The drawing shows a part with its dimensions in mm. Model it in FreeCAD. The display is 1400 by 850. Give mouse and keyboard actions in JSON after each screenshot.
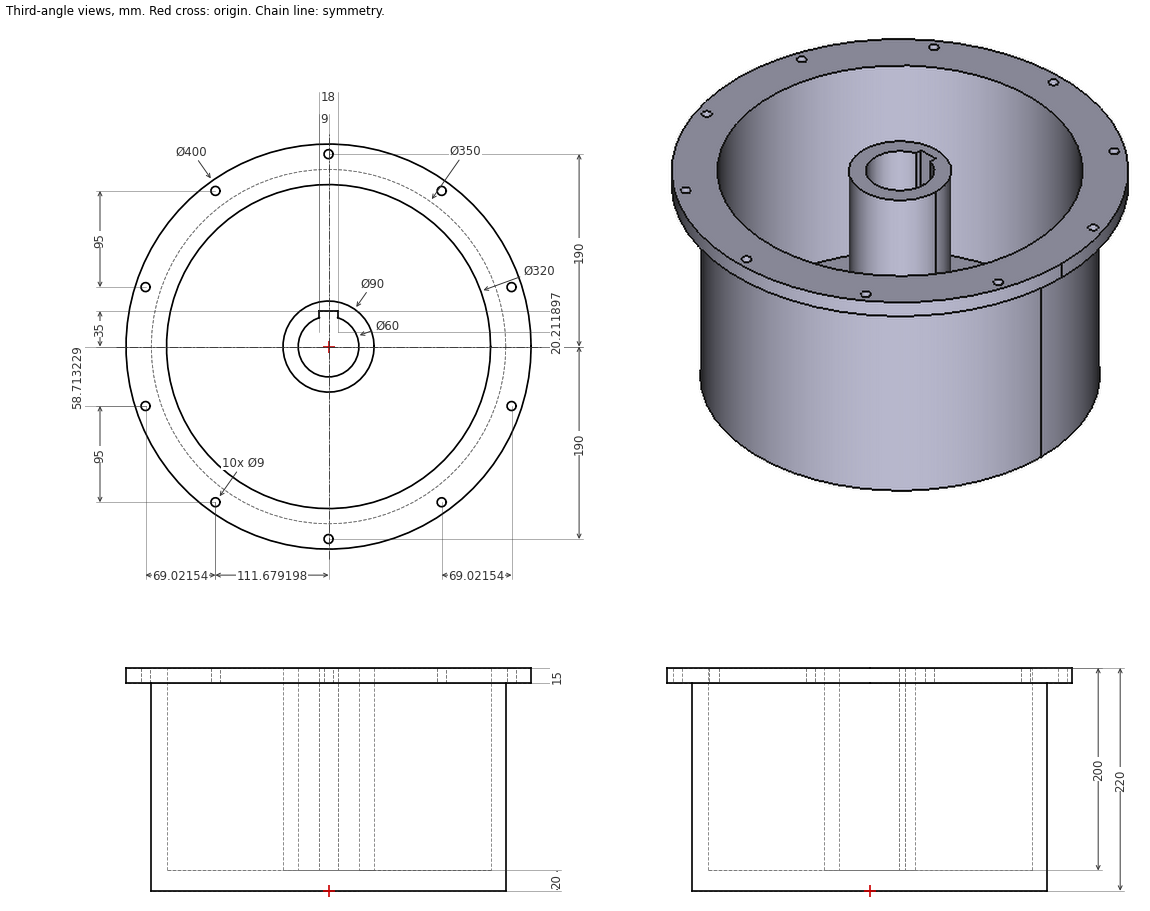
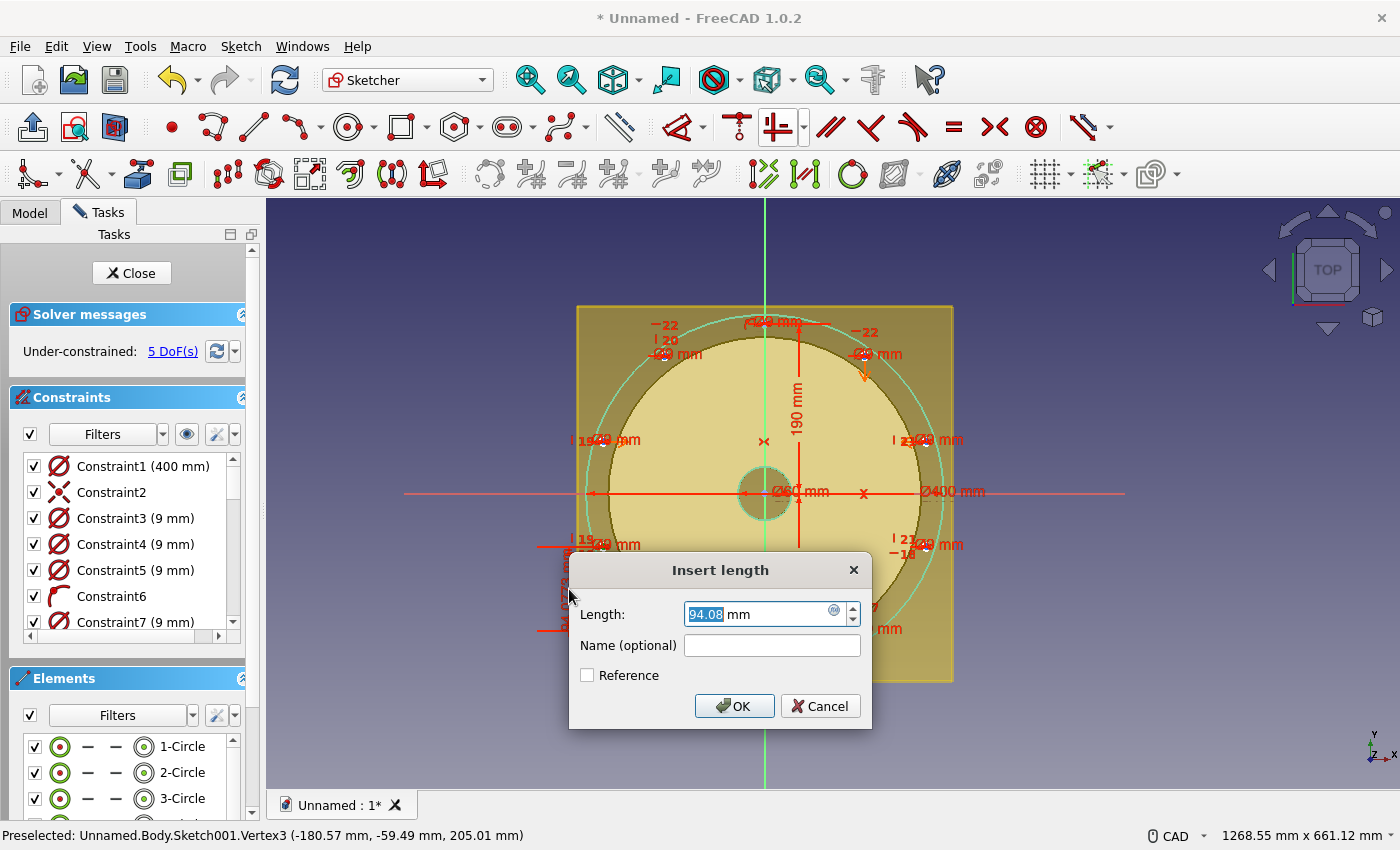
{"action": "type", "text": "95"}
{"action": "key", "text": "Return"}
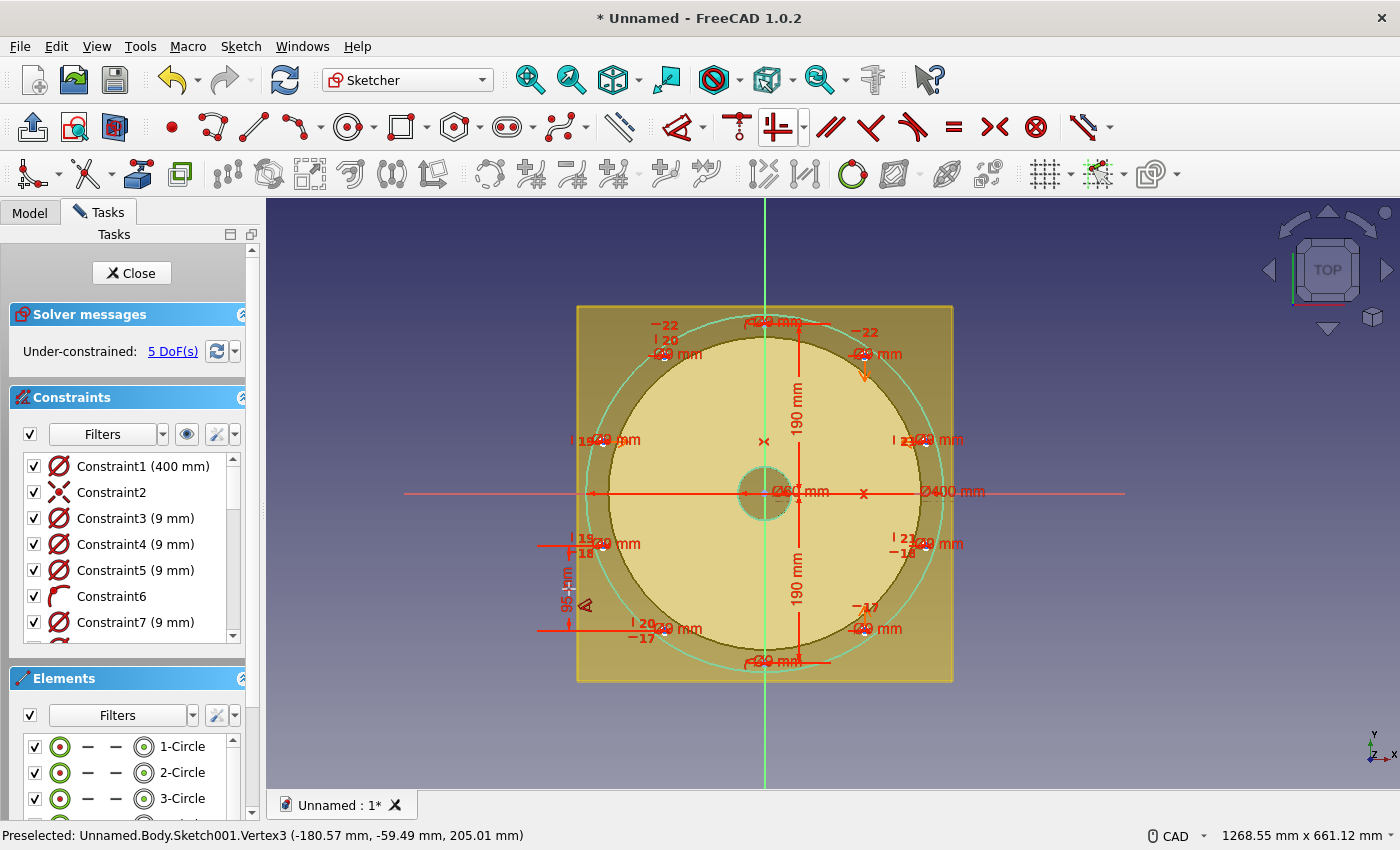
{"action": "left_click", "coordinate": [603, 442]}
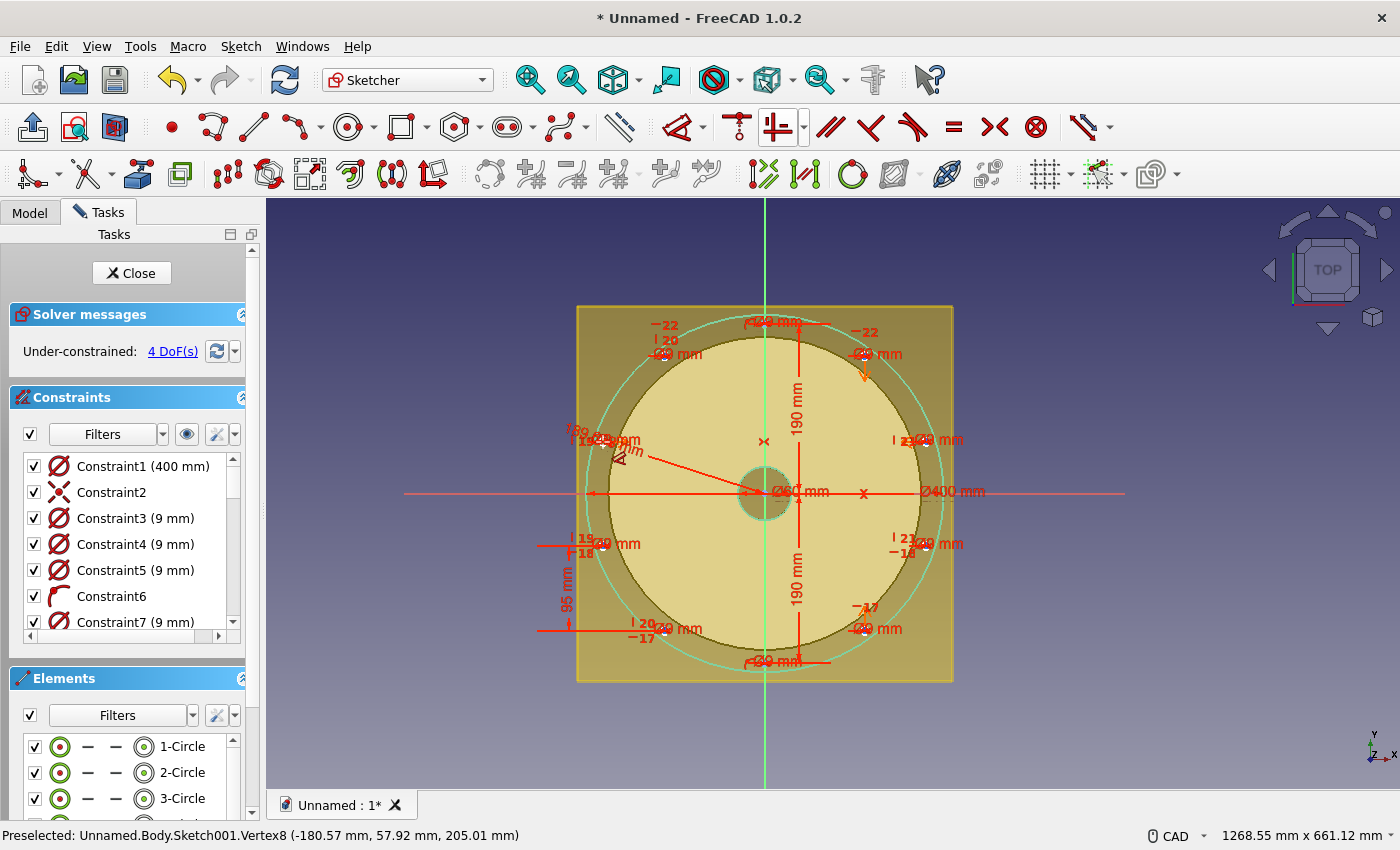
{"action": "left_click", "coordinate": [665, 356]}
{"action": "left_click", "coordinate": [569, 399]}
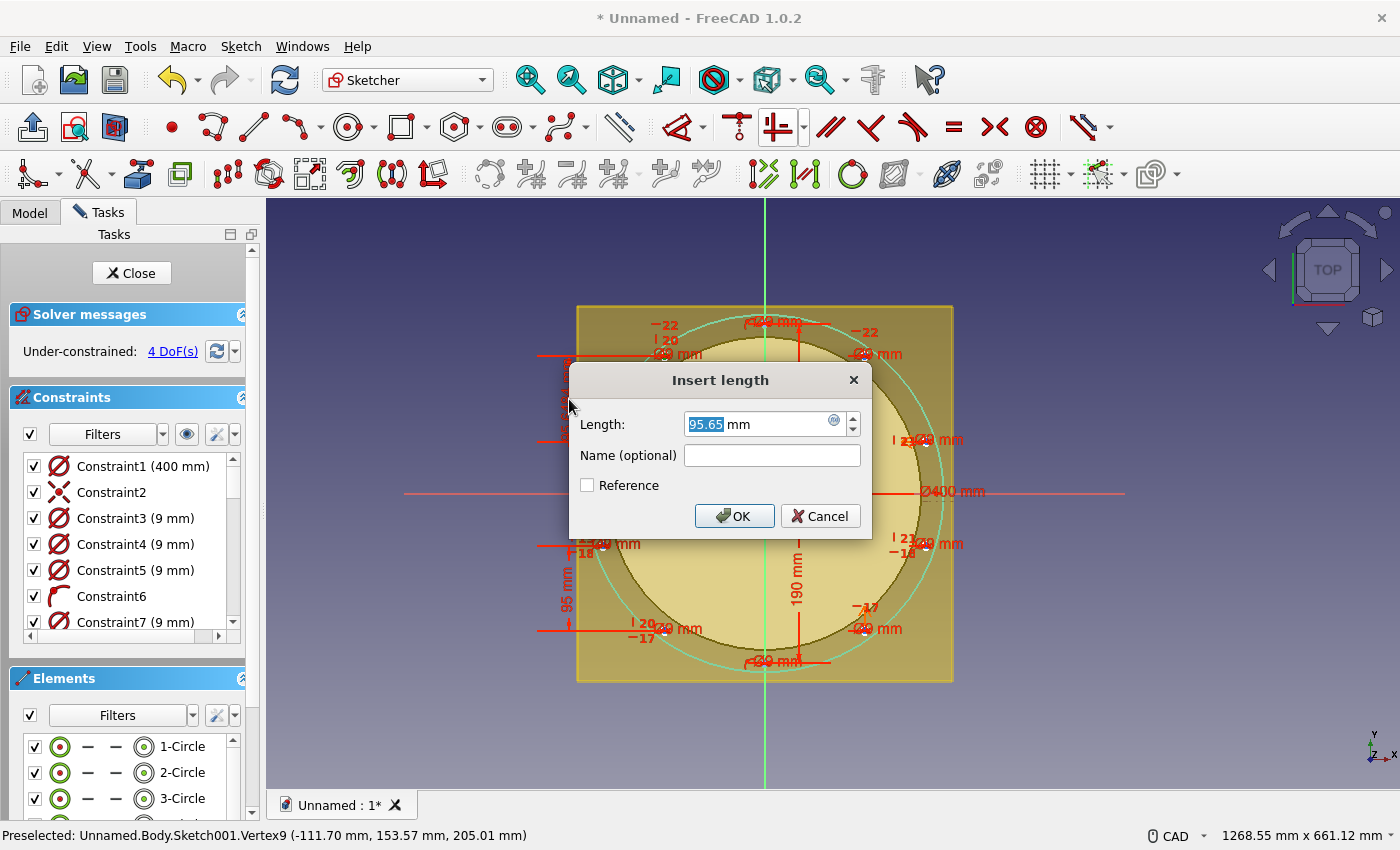
{"action": "type", "text": "95"}
{"action": "key", "text": "Return"}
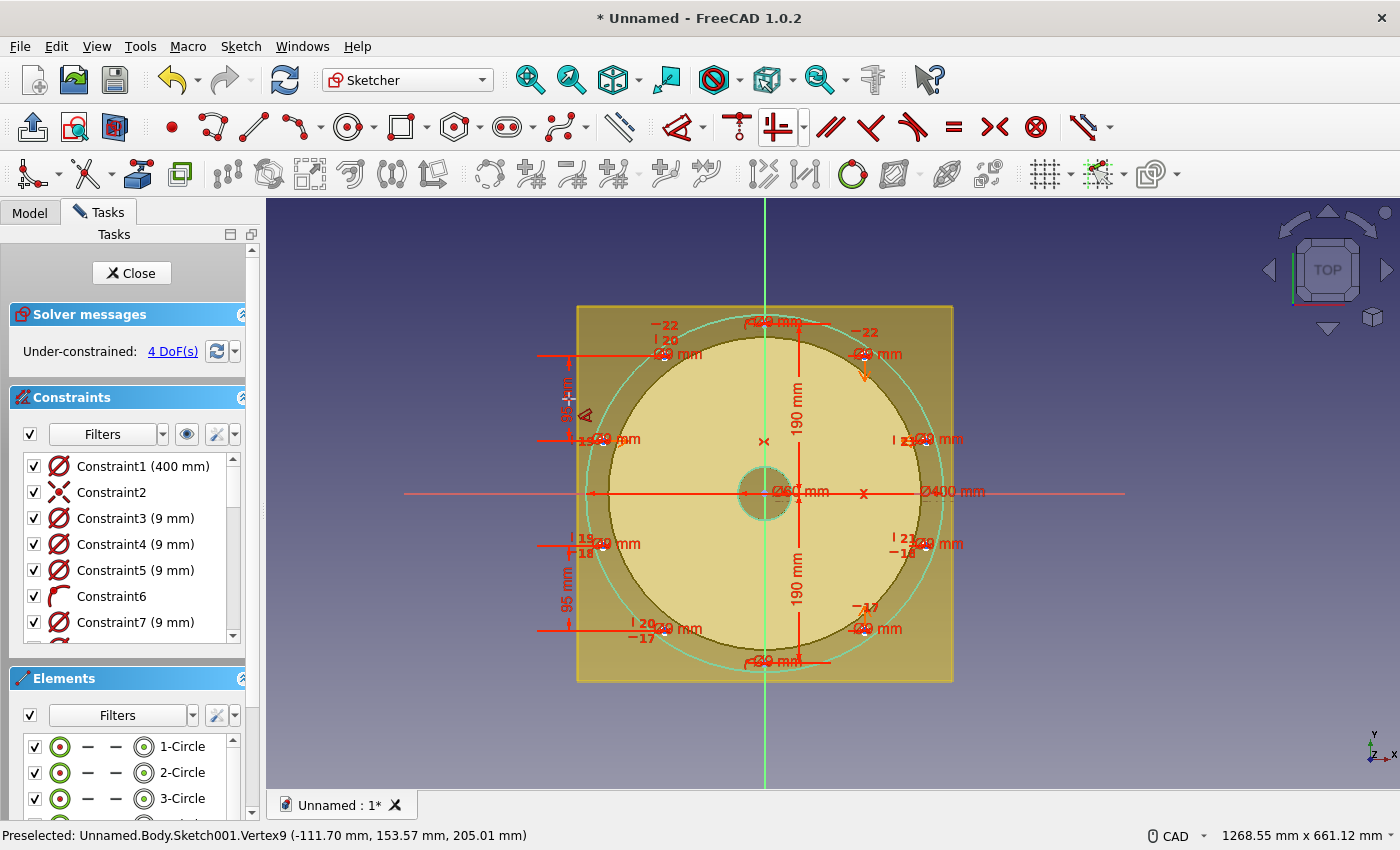
{"action": "left_click", "coordinate": [603, 546]}
{"action": "left_click", "coordinate": [569, 520]}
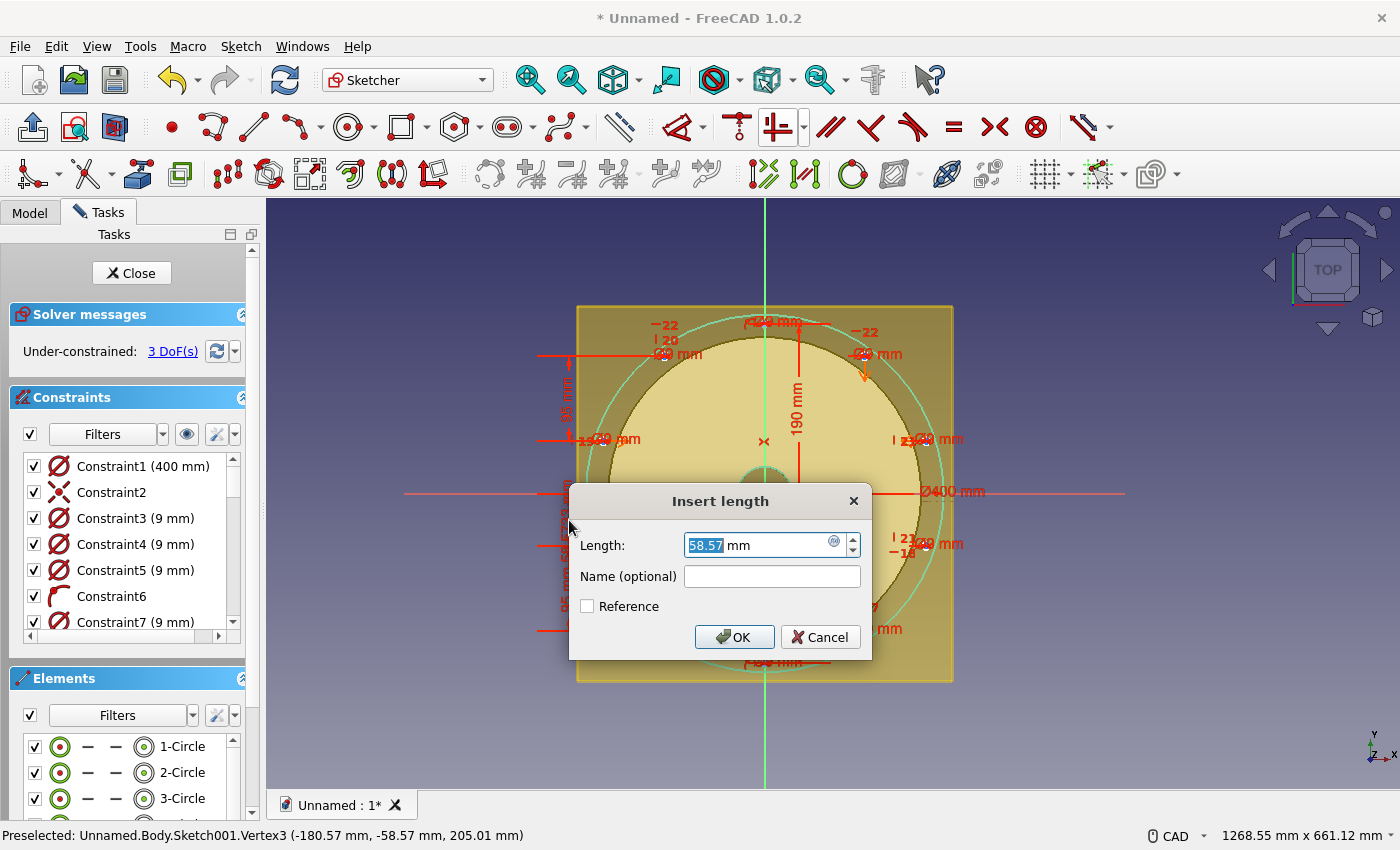
{"action": "type", "text": "58.713229"}
{"action": "key", "text": "Return"}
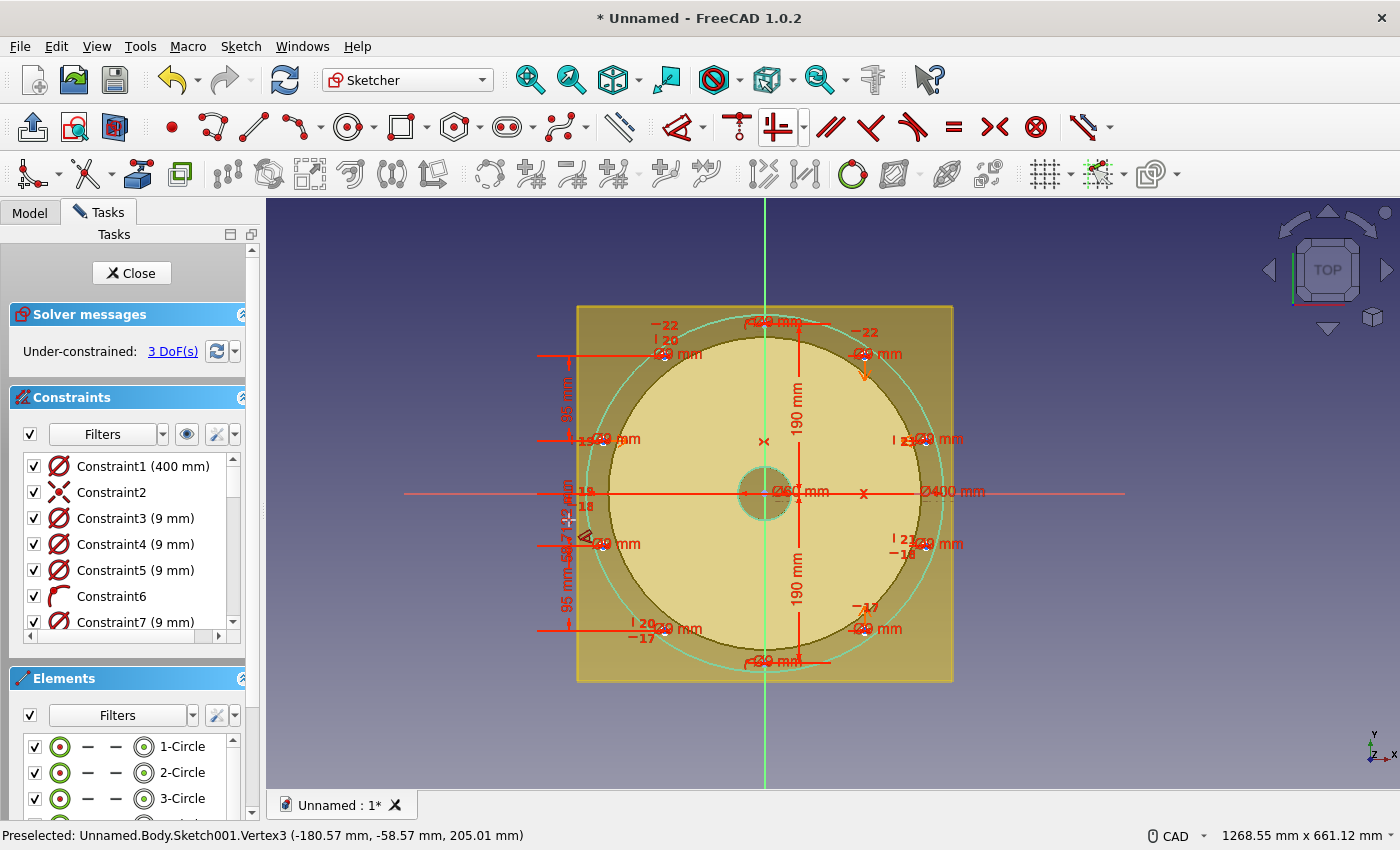
{"action": "left_click", "coordinate": [665, 631]}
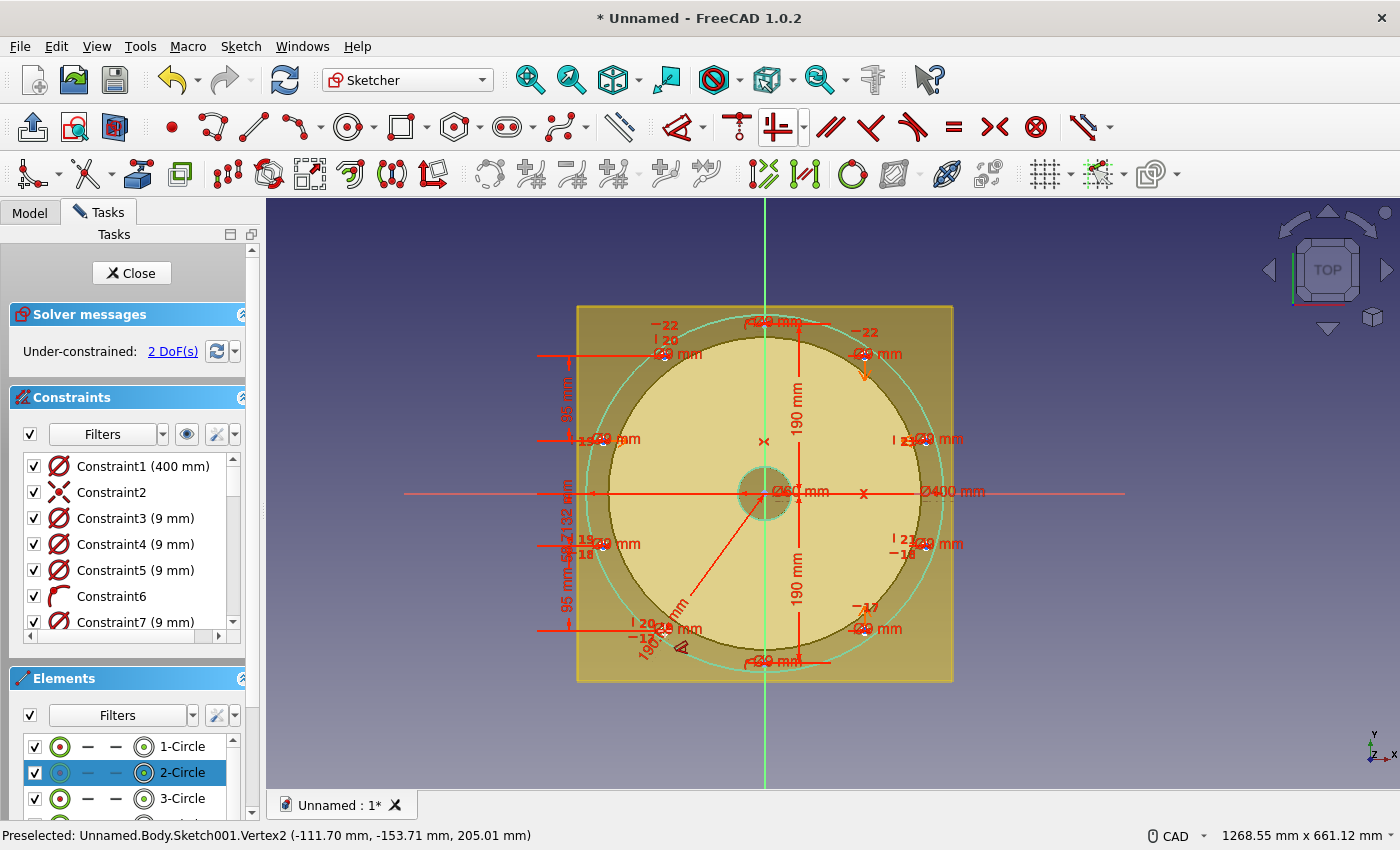
{"action": "left_click", "coordinate": [603, 546]}
{"action": "left_click", "coordinate": [634, 665]}